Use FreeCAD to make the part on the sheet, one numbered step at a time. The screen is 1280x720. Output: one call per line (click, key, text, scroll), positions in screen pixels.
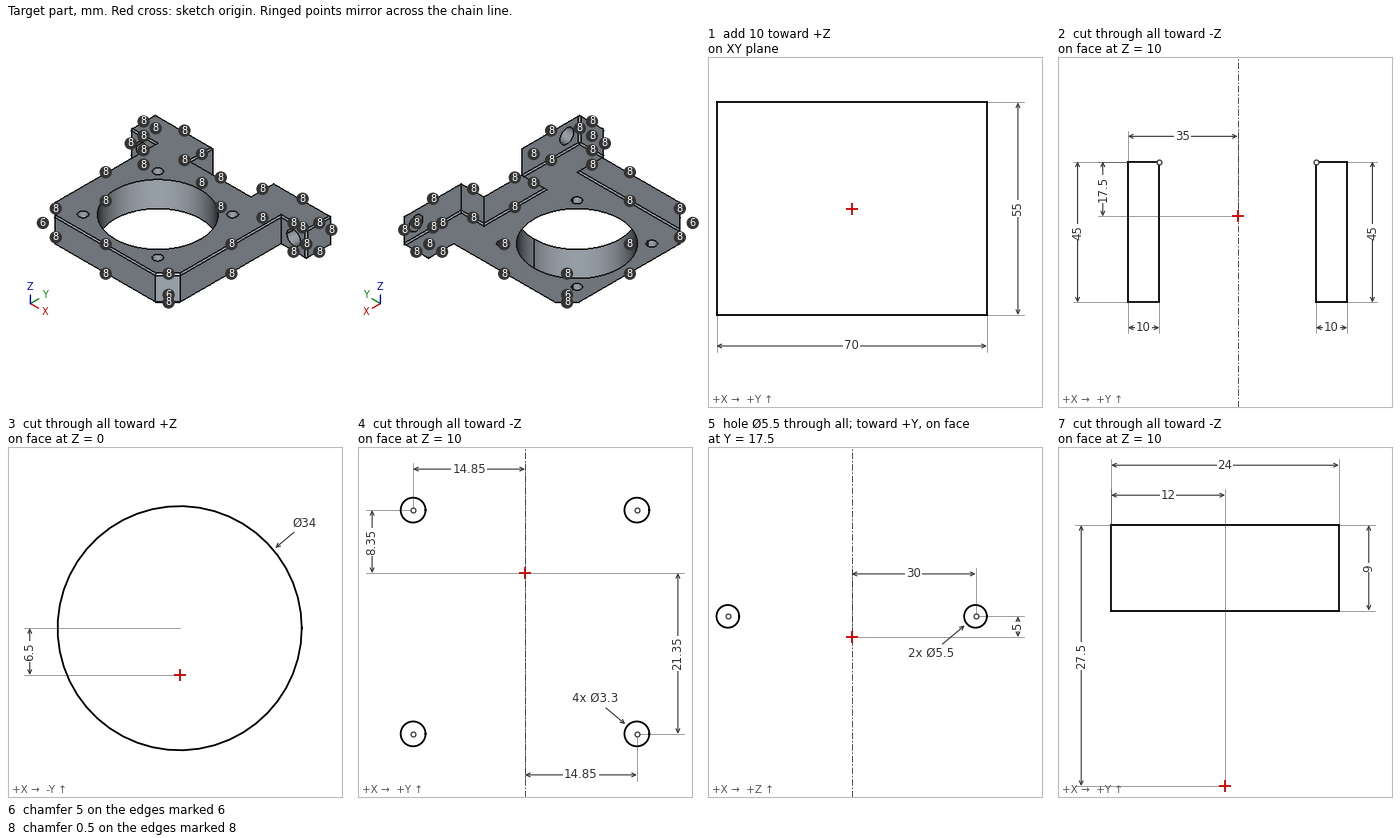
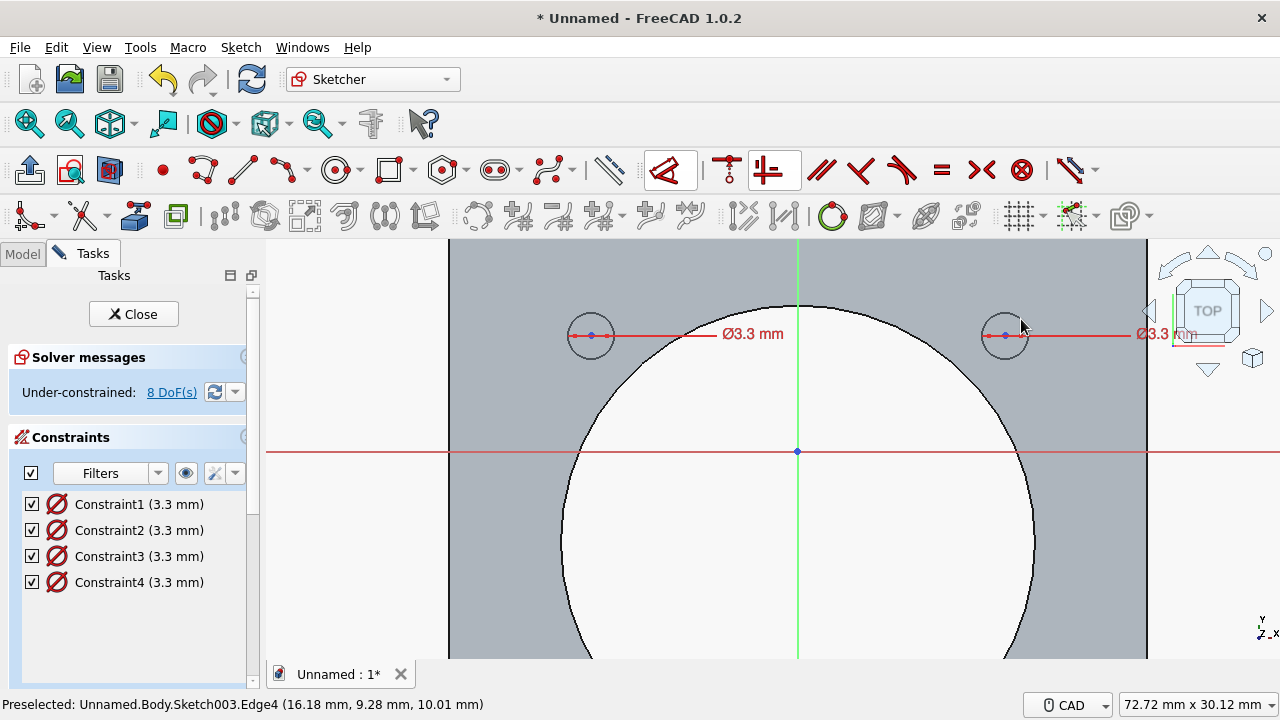
scroll(591, 335, down, 3)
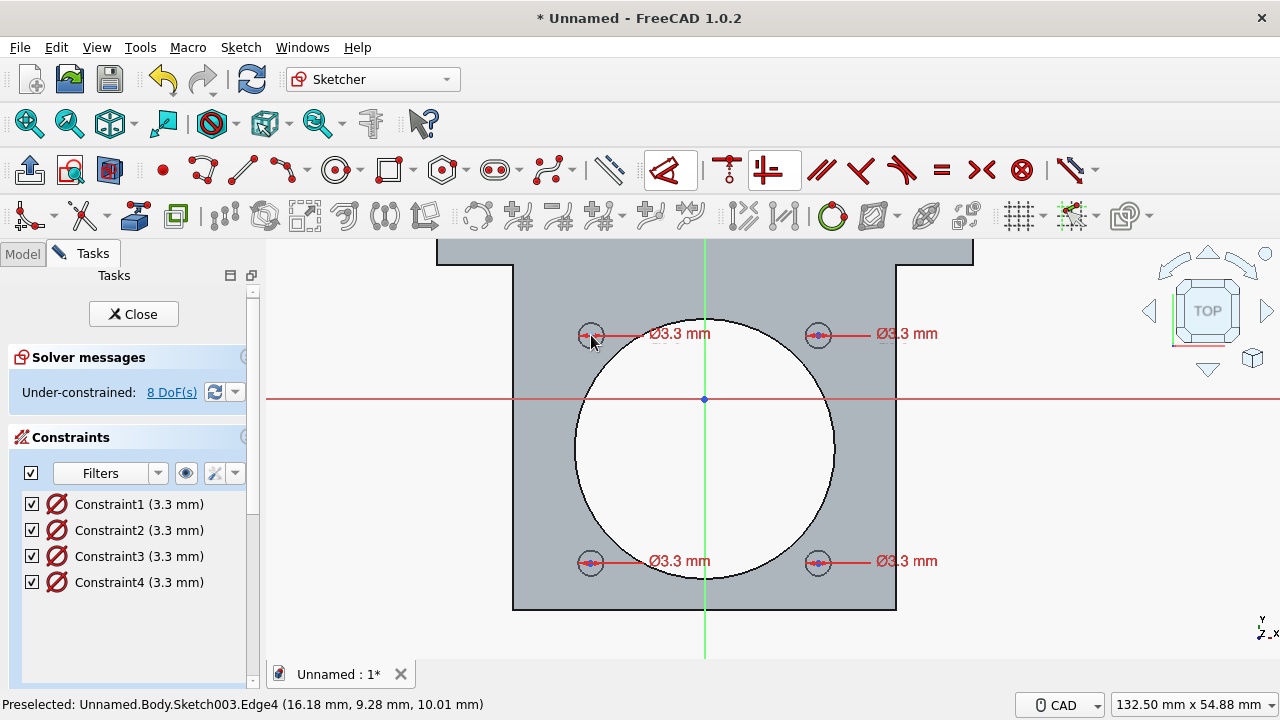
click(818, 563)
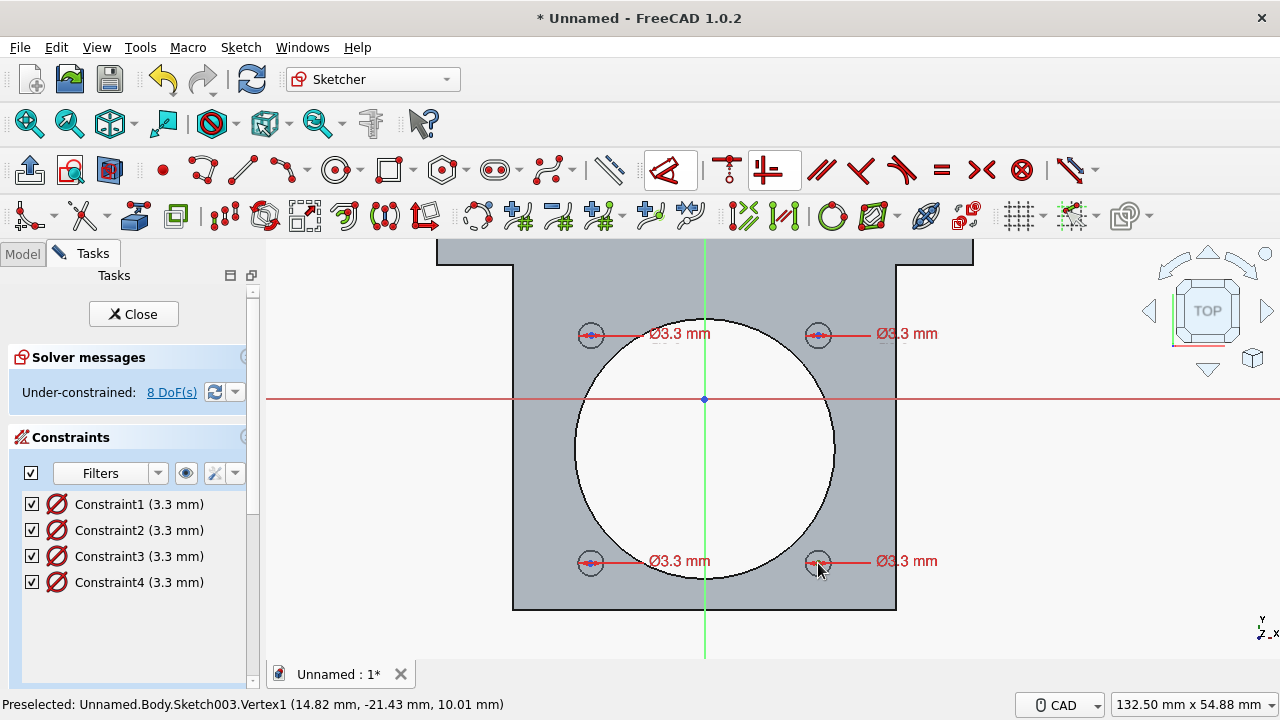
click(591, 563)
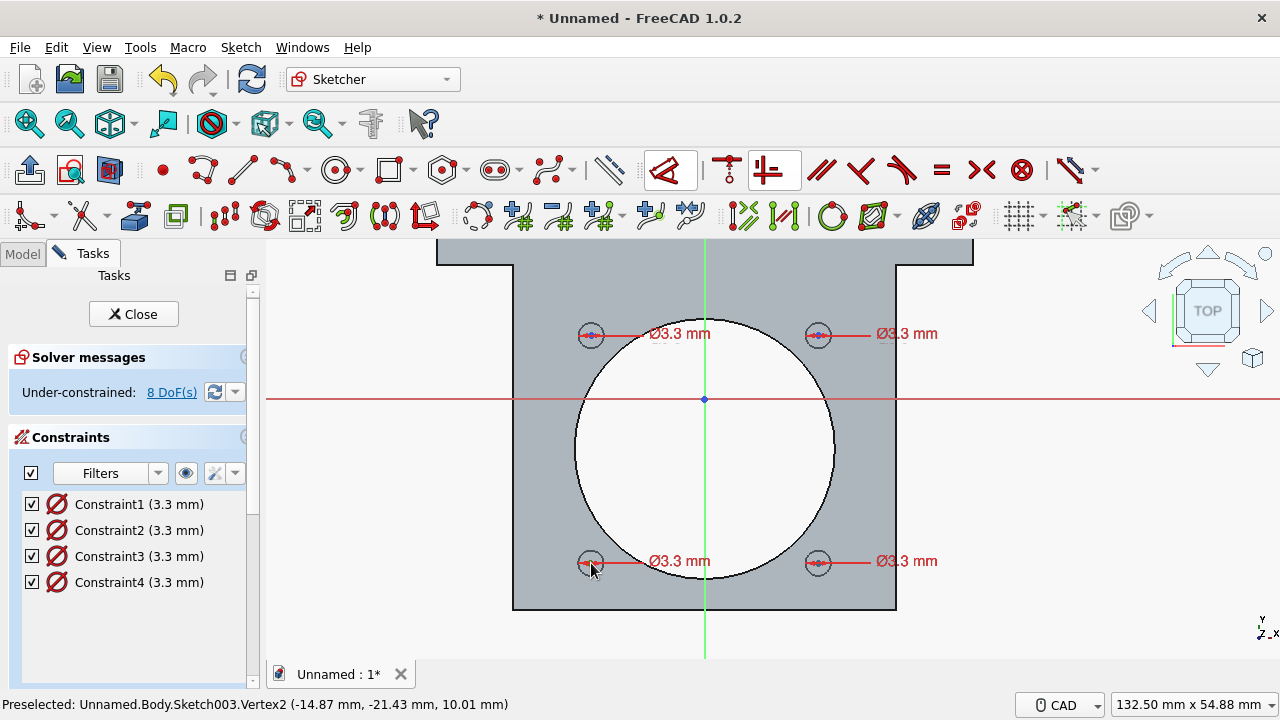
click(705, 605)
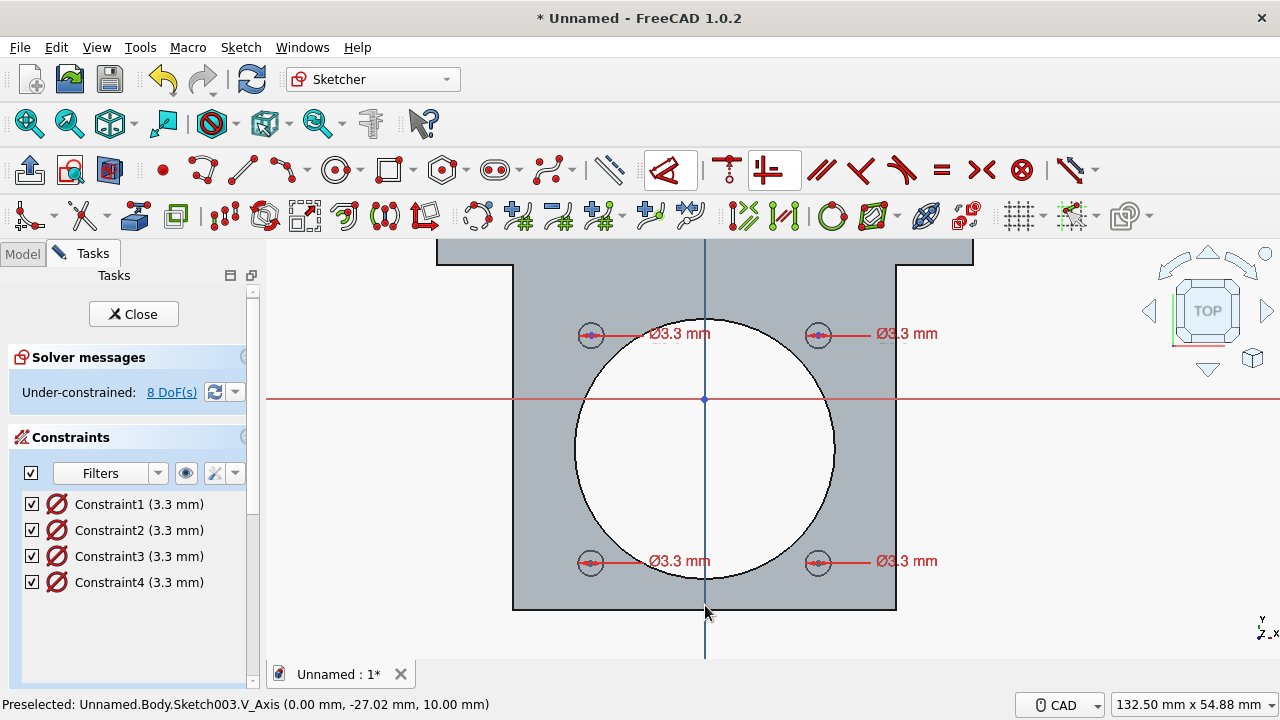
key(s)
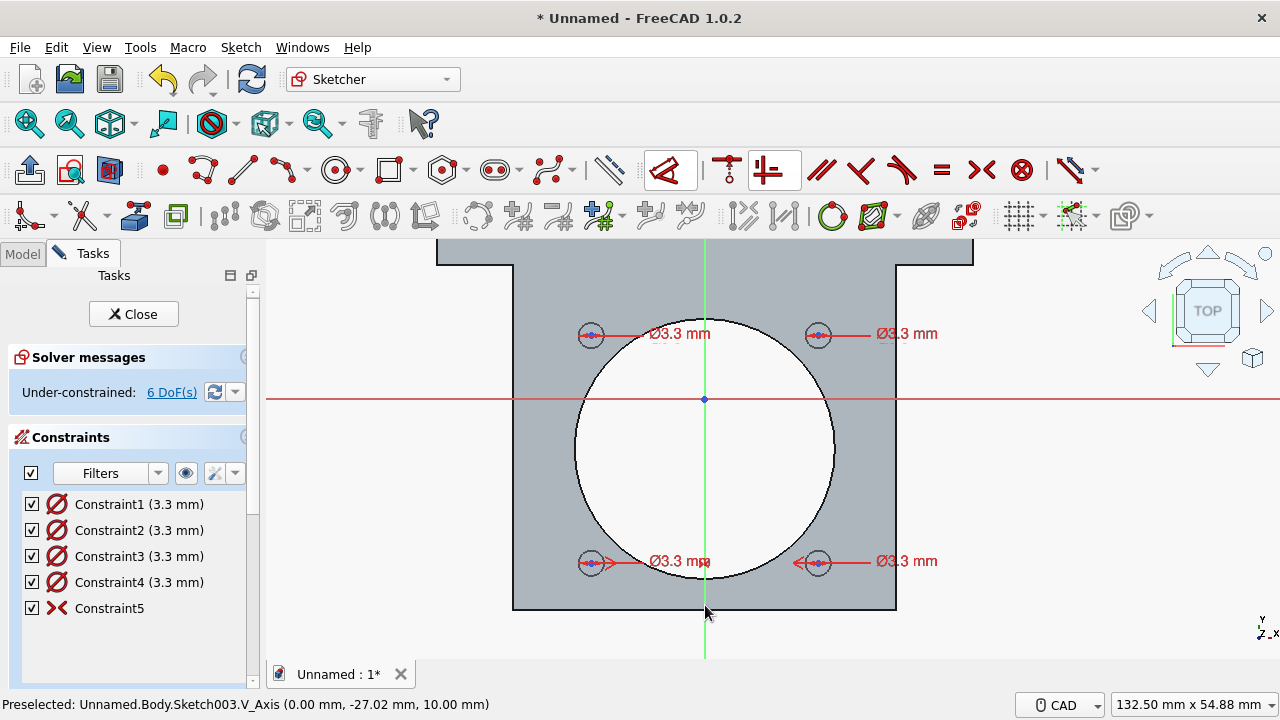
click(591, 336)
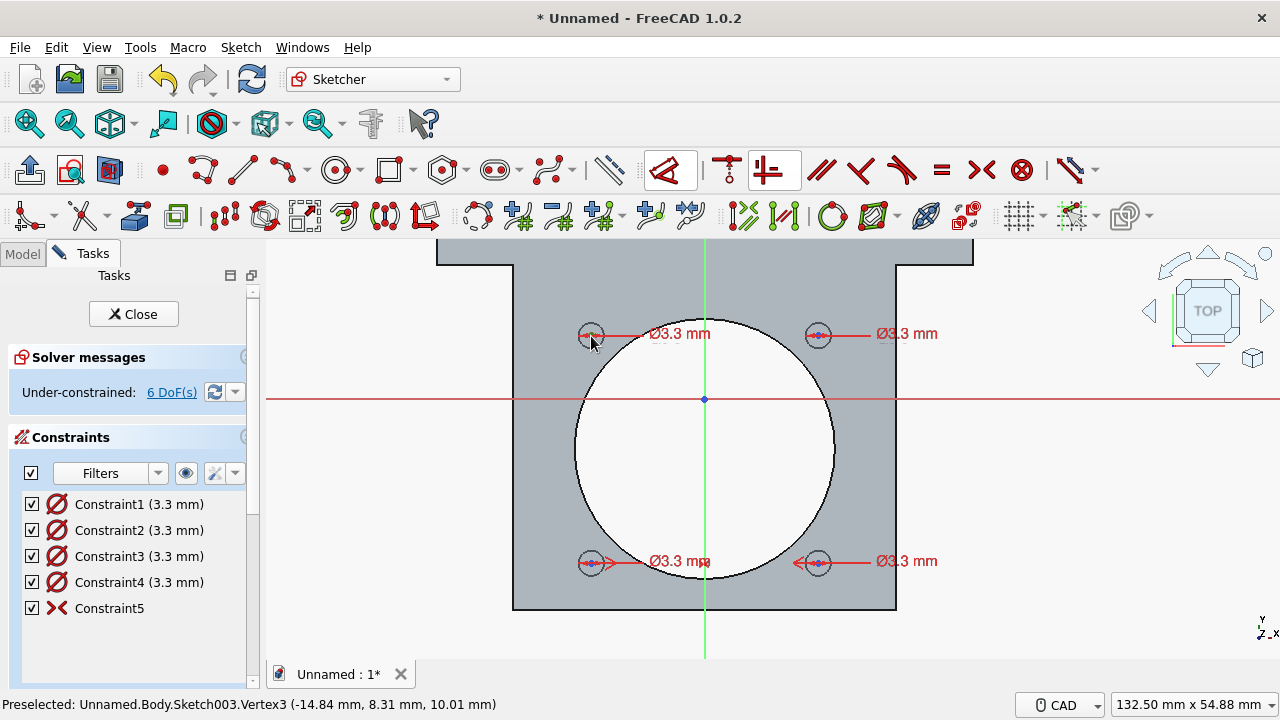
click(818, 336)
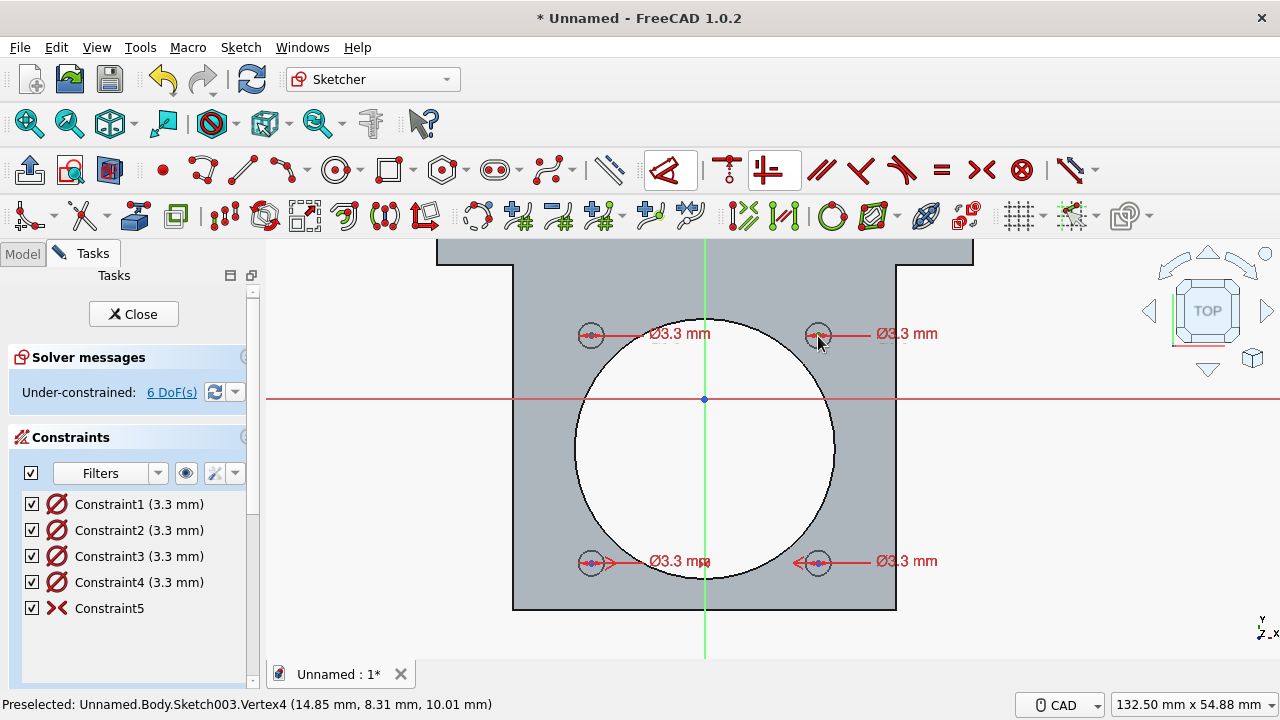
click(705, 605)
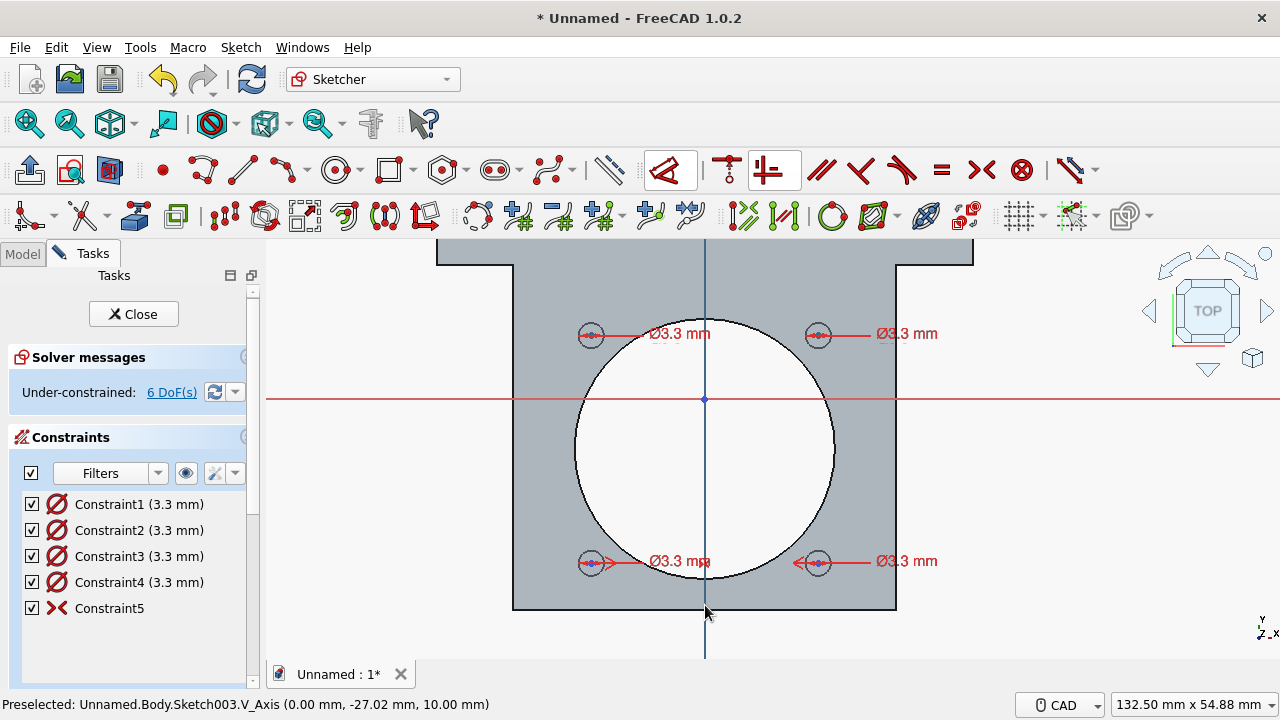
key(s)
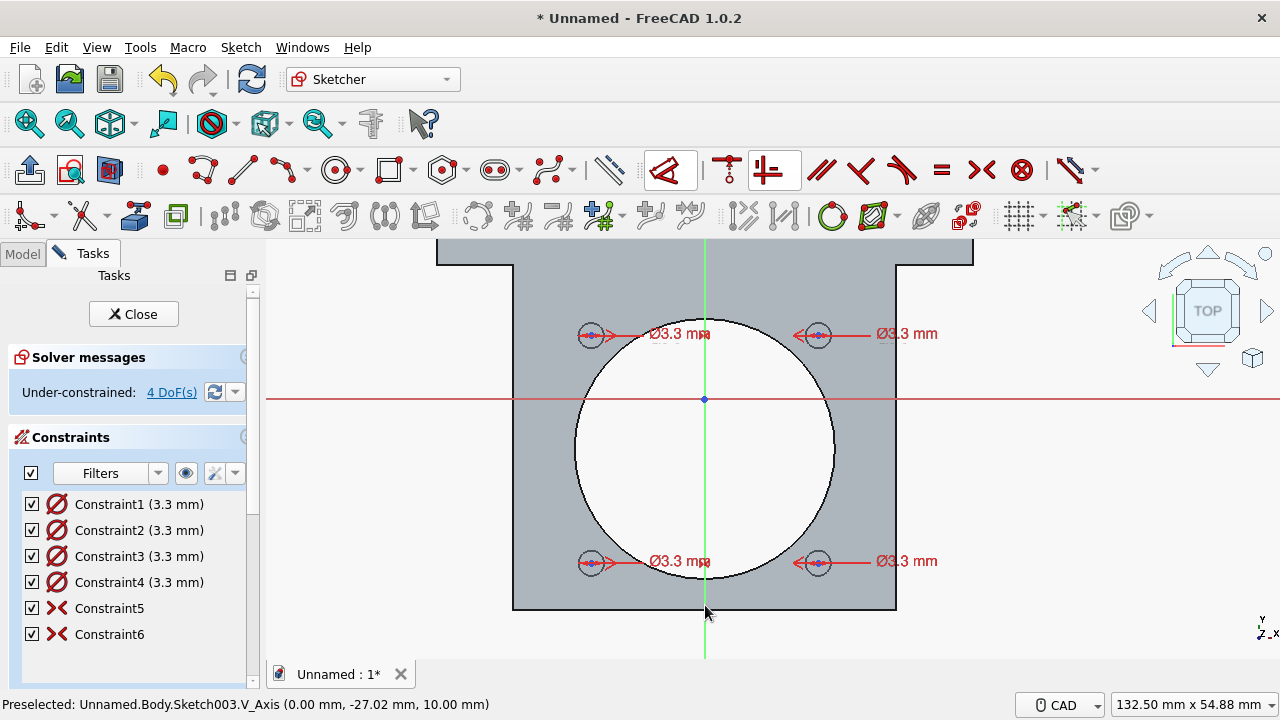
click(591, 336)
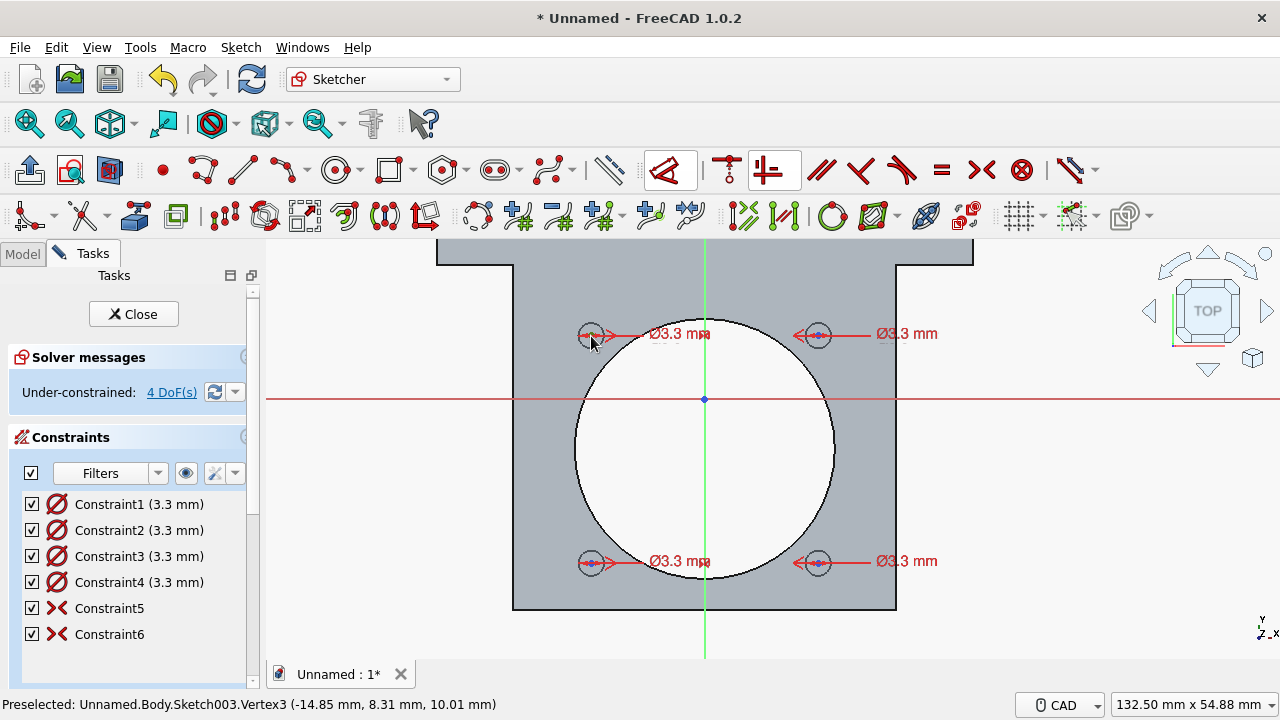
key(i)